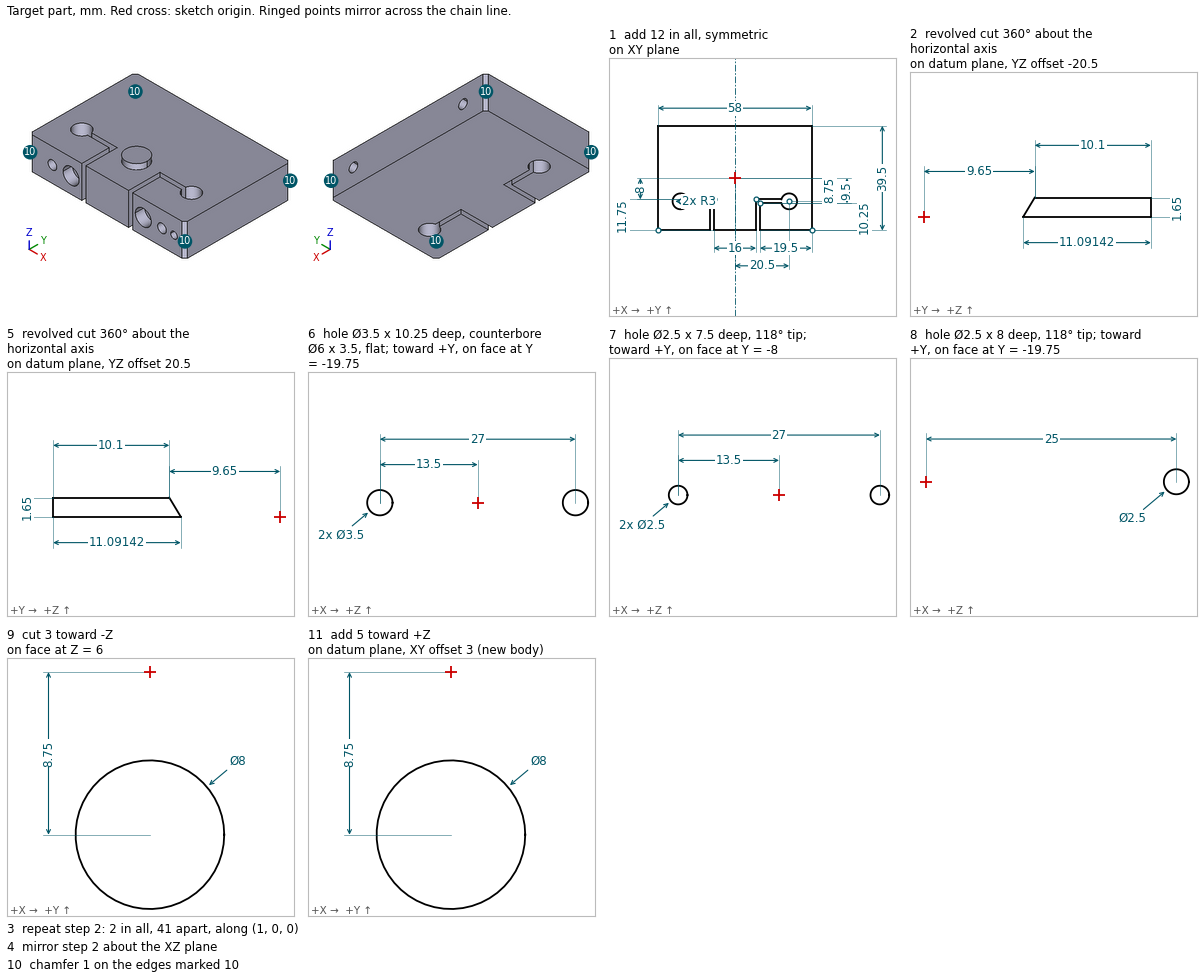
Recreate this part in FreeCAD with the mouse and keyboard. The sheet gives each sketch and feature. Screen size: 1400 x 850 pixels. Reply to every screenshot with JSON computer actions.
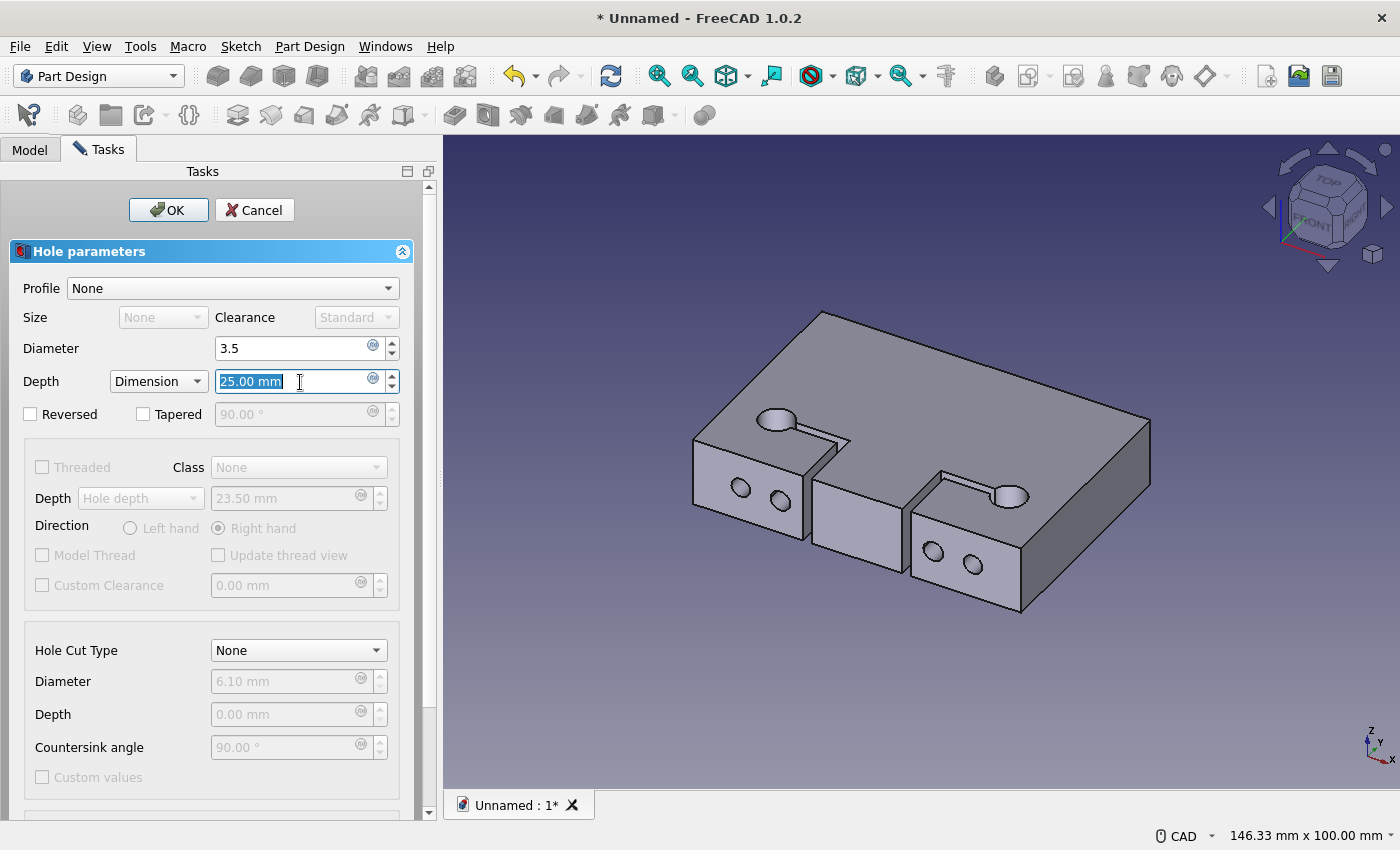
{"action": "type", "text": "10.25"}
{"action": "key", "text": "Tab"}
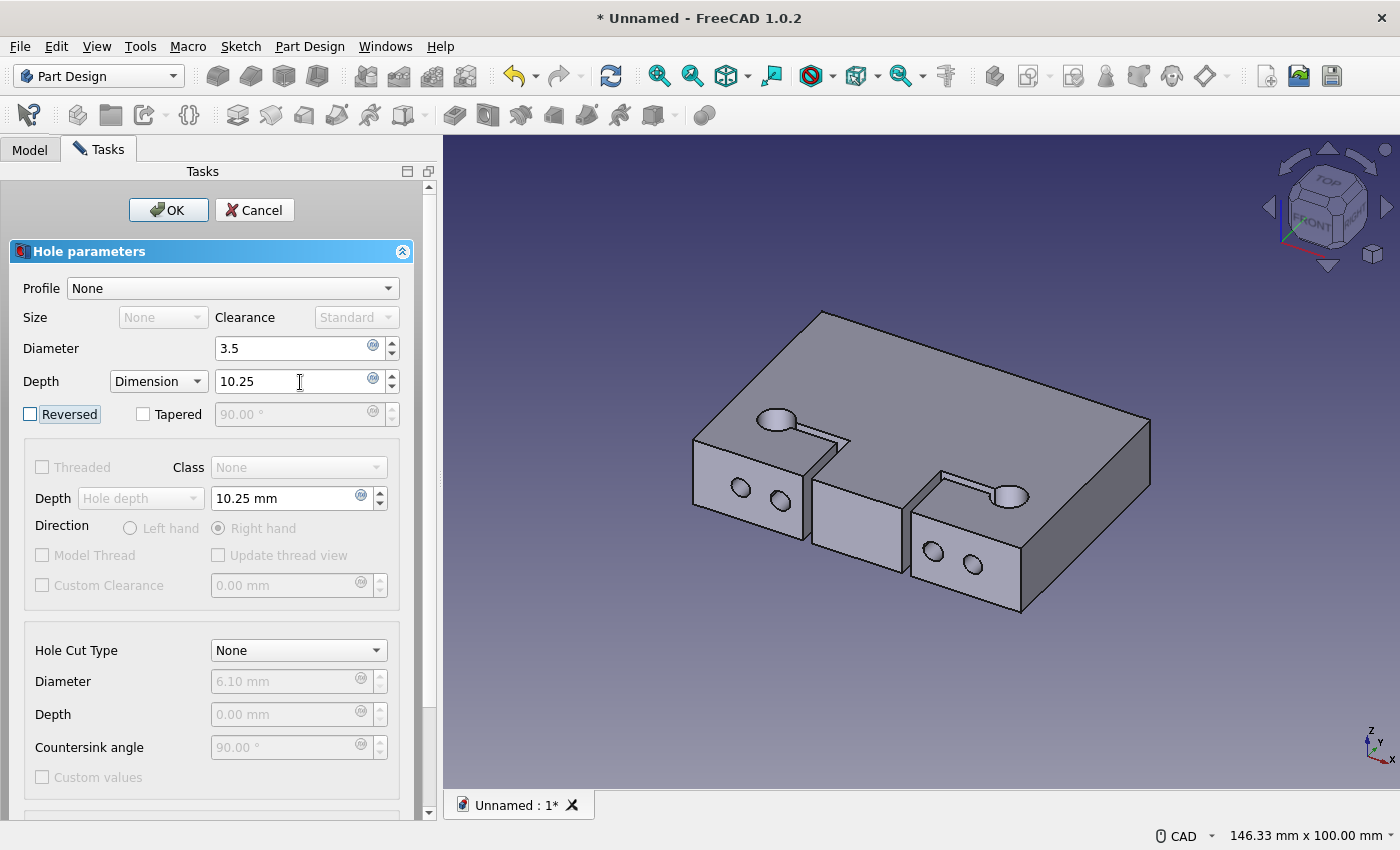
{"action": "left_click", "coordinate": [300, 650]}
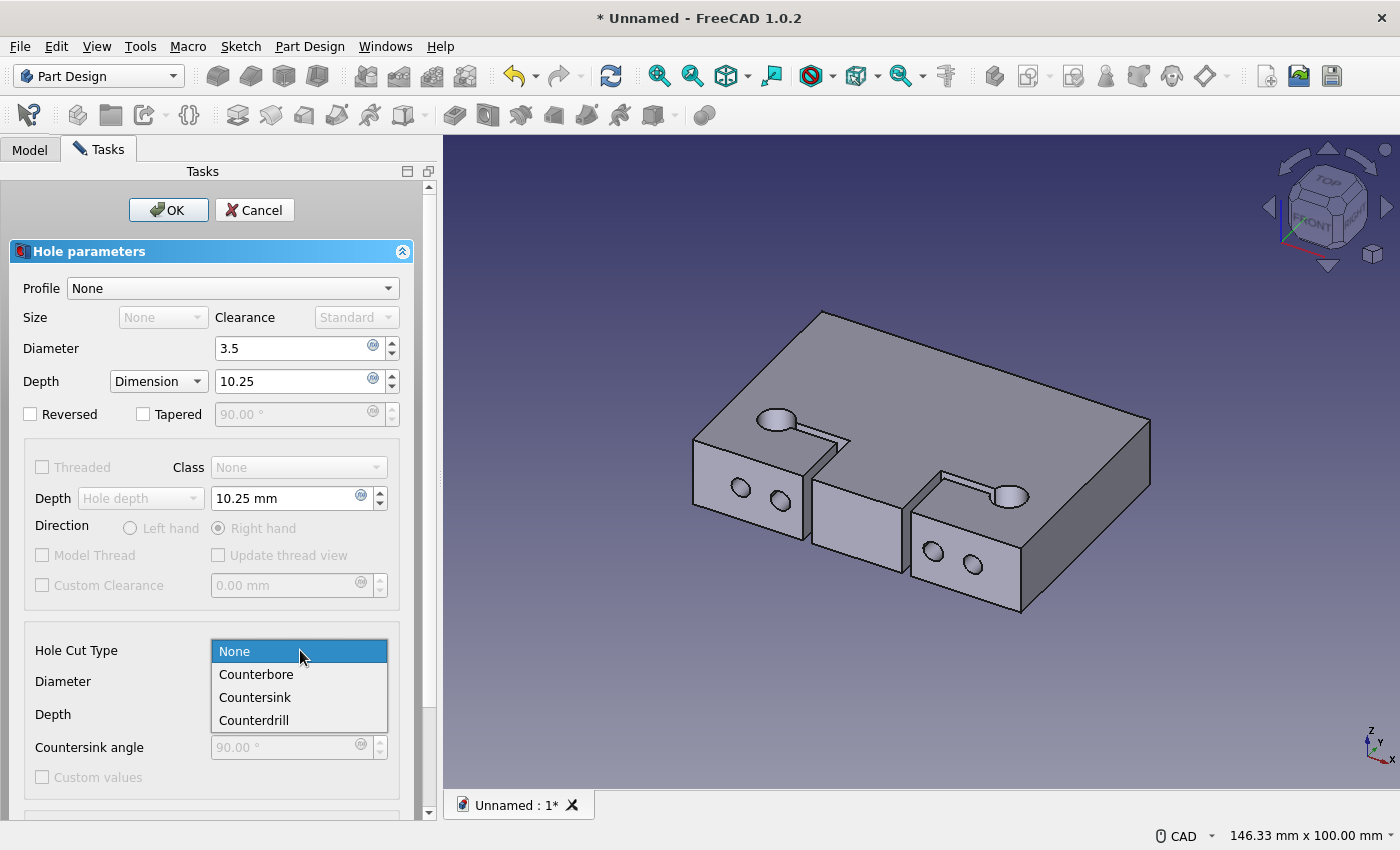
{"action": "left_click", "coordinate": [298, 674]}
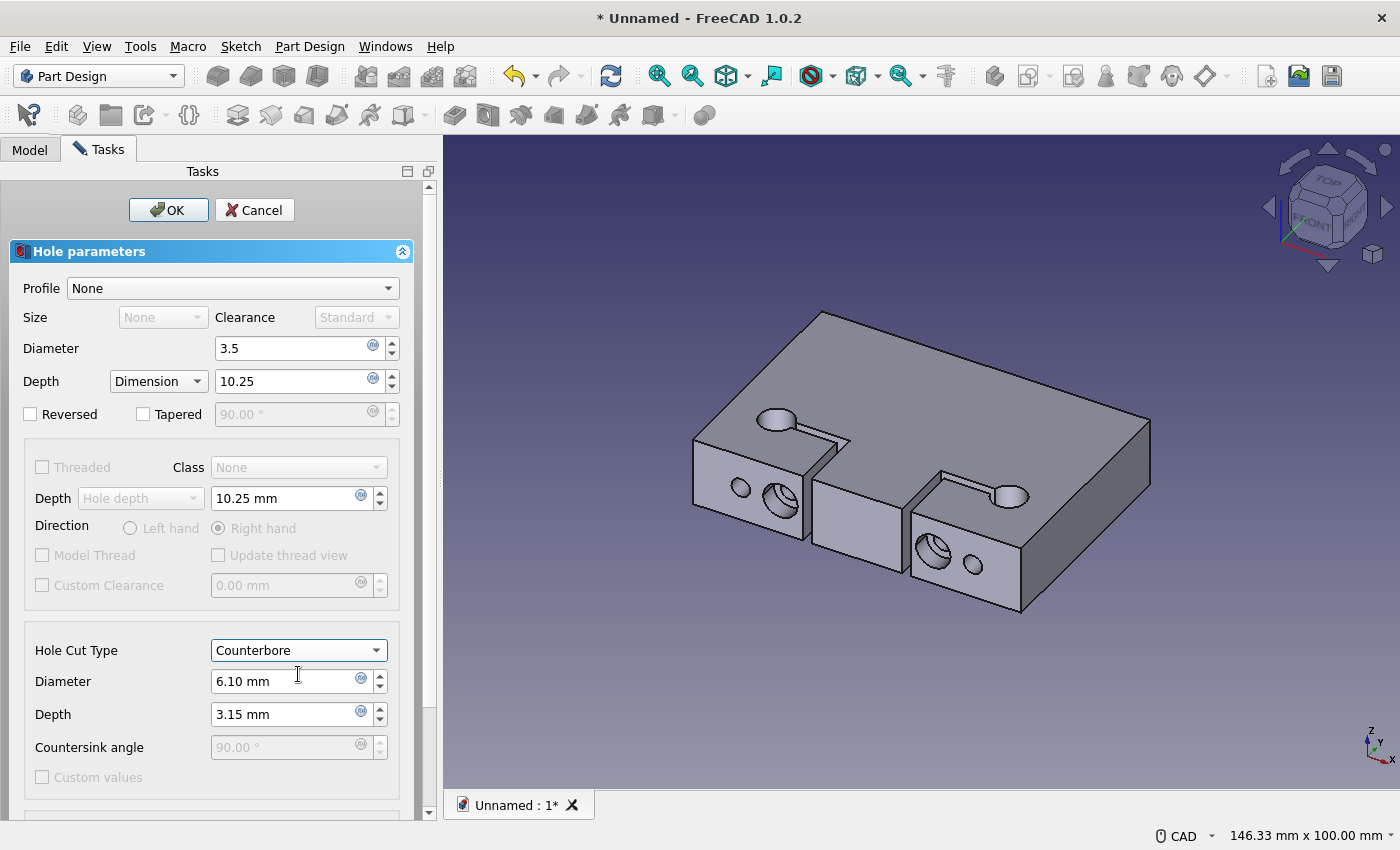
{"action": "triple_click", "coordinate": [292, 682]}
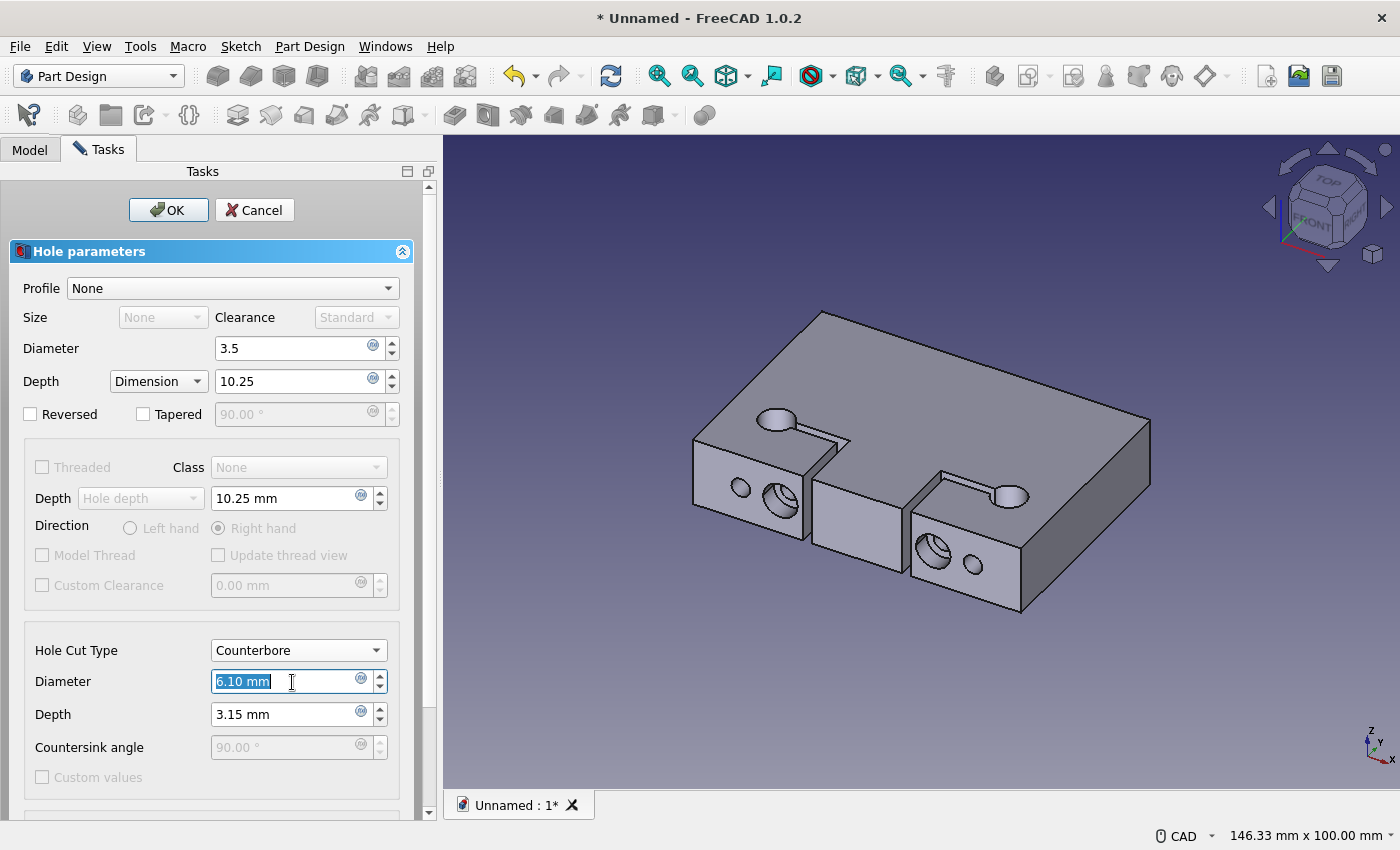
{"action": "type", "text": "6"}
{"action": "key", "text": "Tab"}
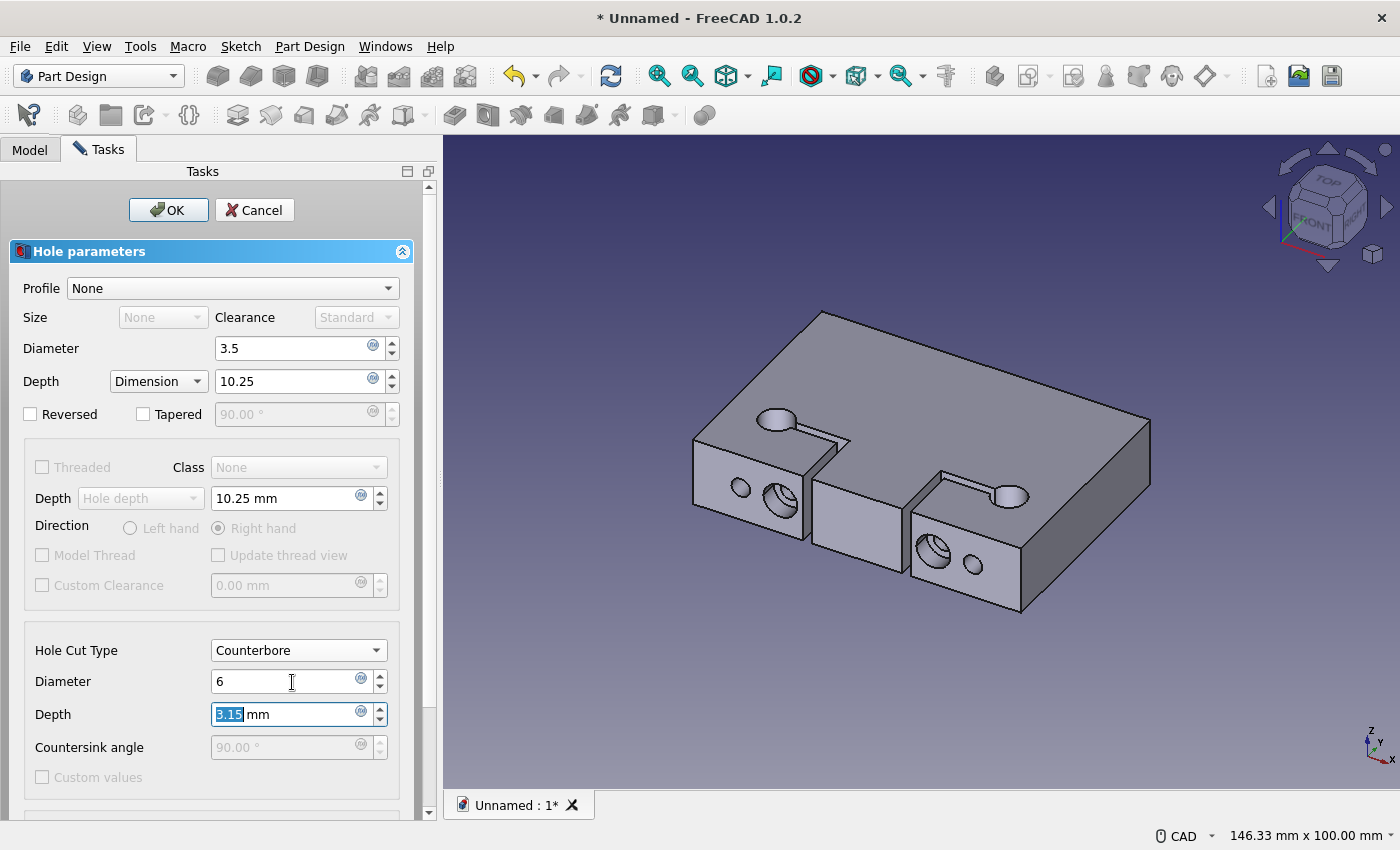
{"action": "type", "text": "3.5"}
{"action": "key", "text": "Tab"}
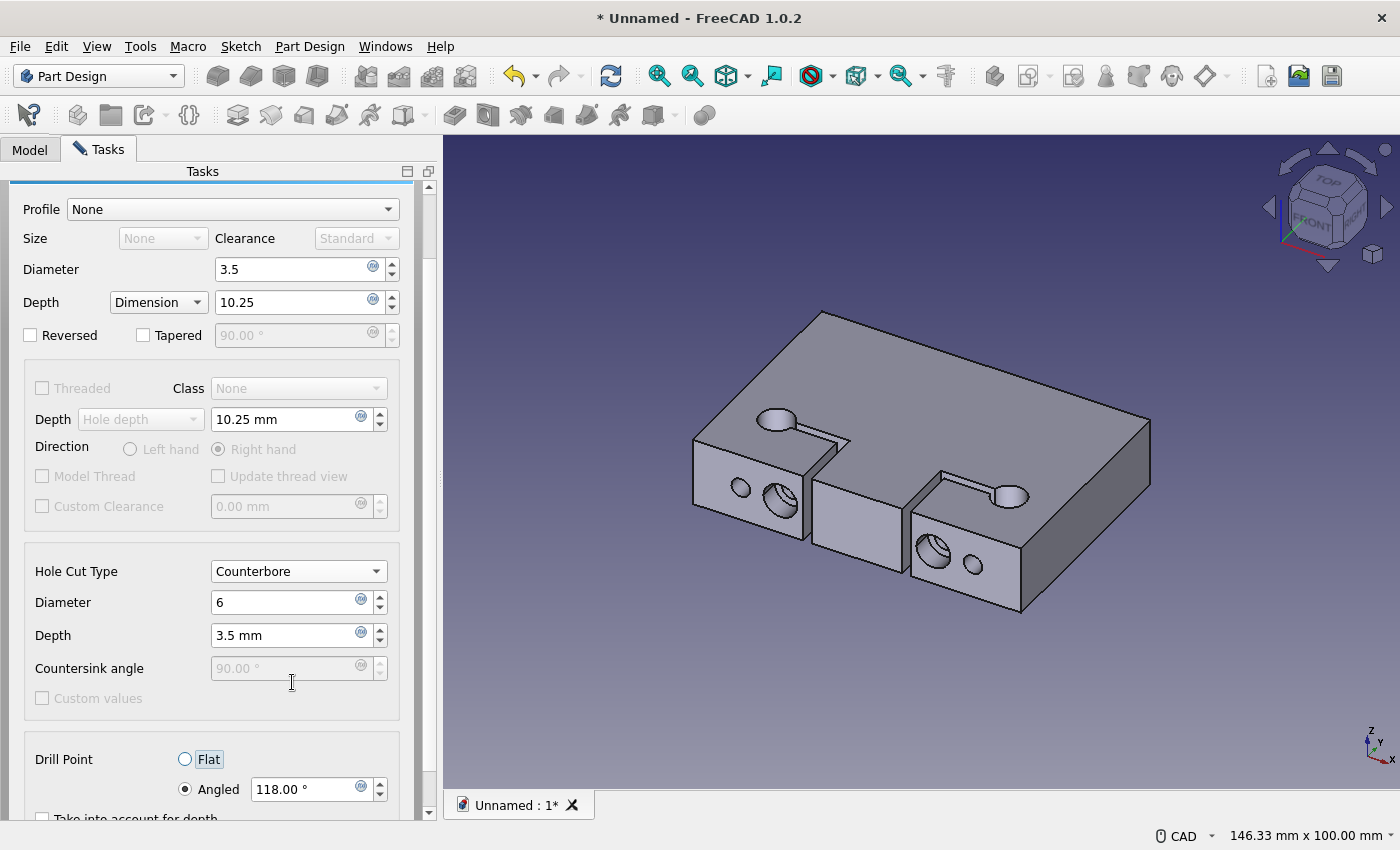
{"action": "left_click", "coordinate": [186, 757]}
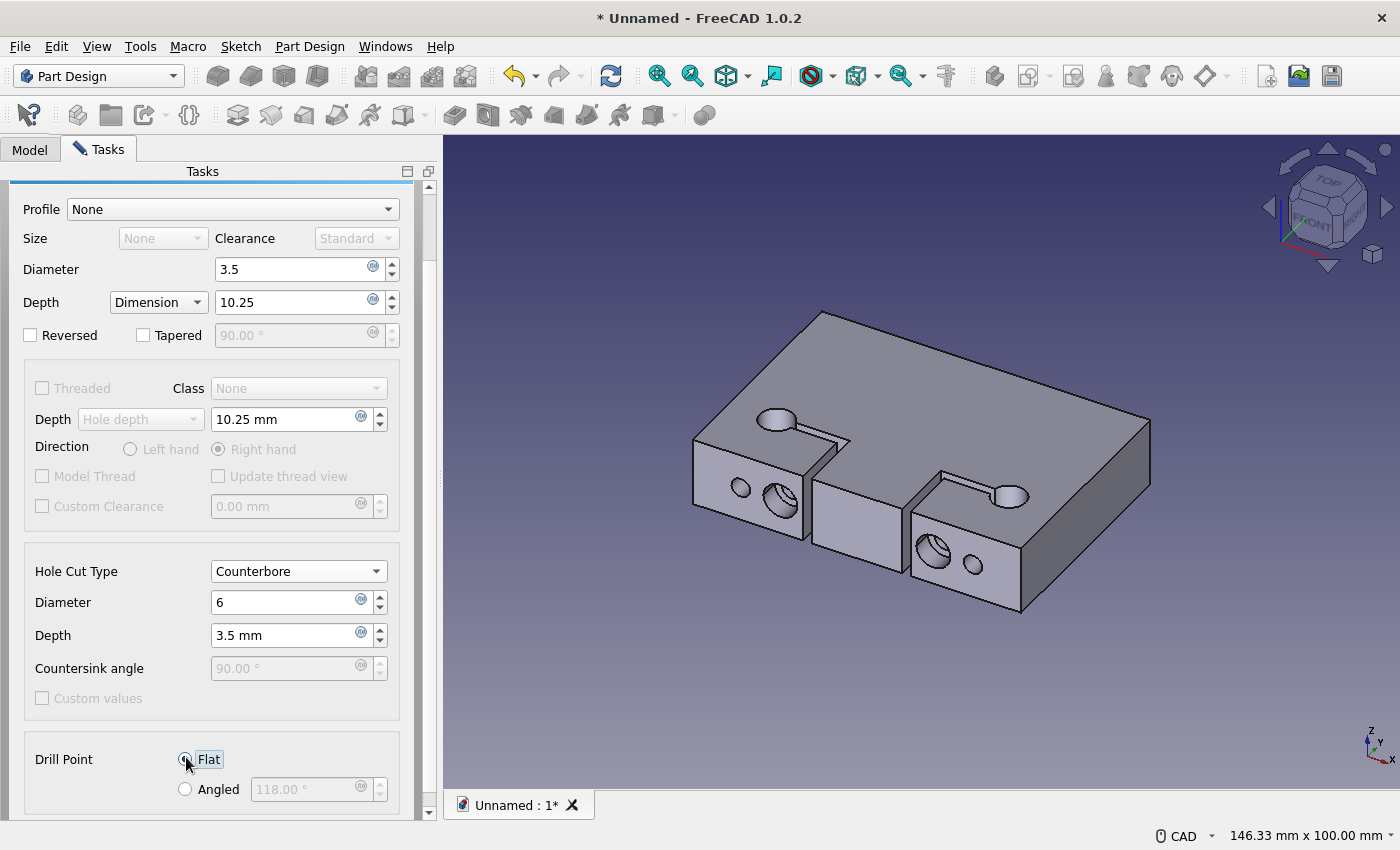
{"action": "scroll", "coordinate": [429, 500], "scroll_direction": "up", "scroll_amount": 3}